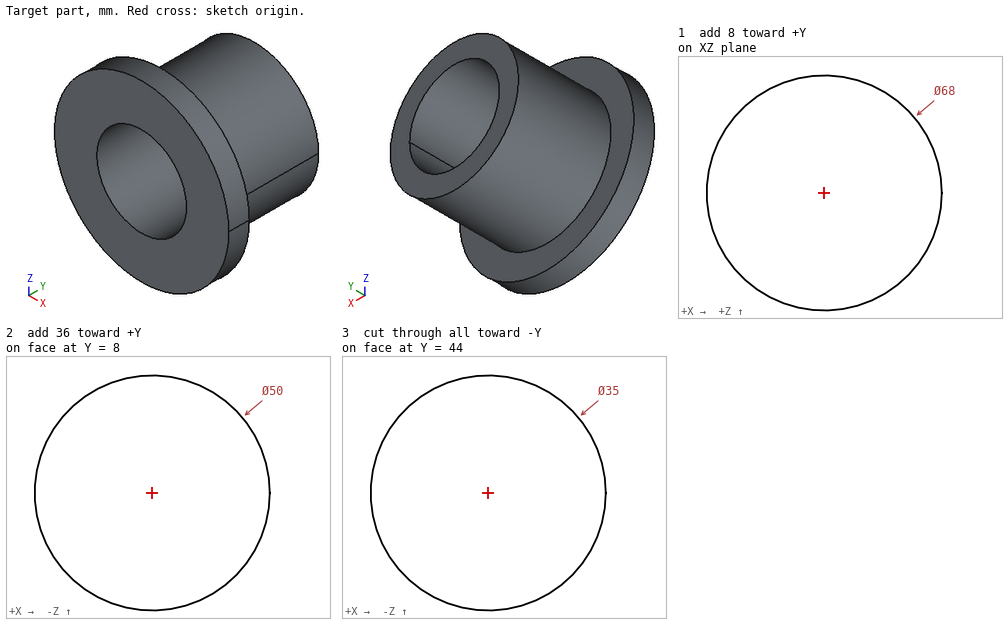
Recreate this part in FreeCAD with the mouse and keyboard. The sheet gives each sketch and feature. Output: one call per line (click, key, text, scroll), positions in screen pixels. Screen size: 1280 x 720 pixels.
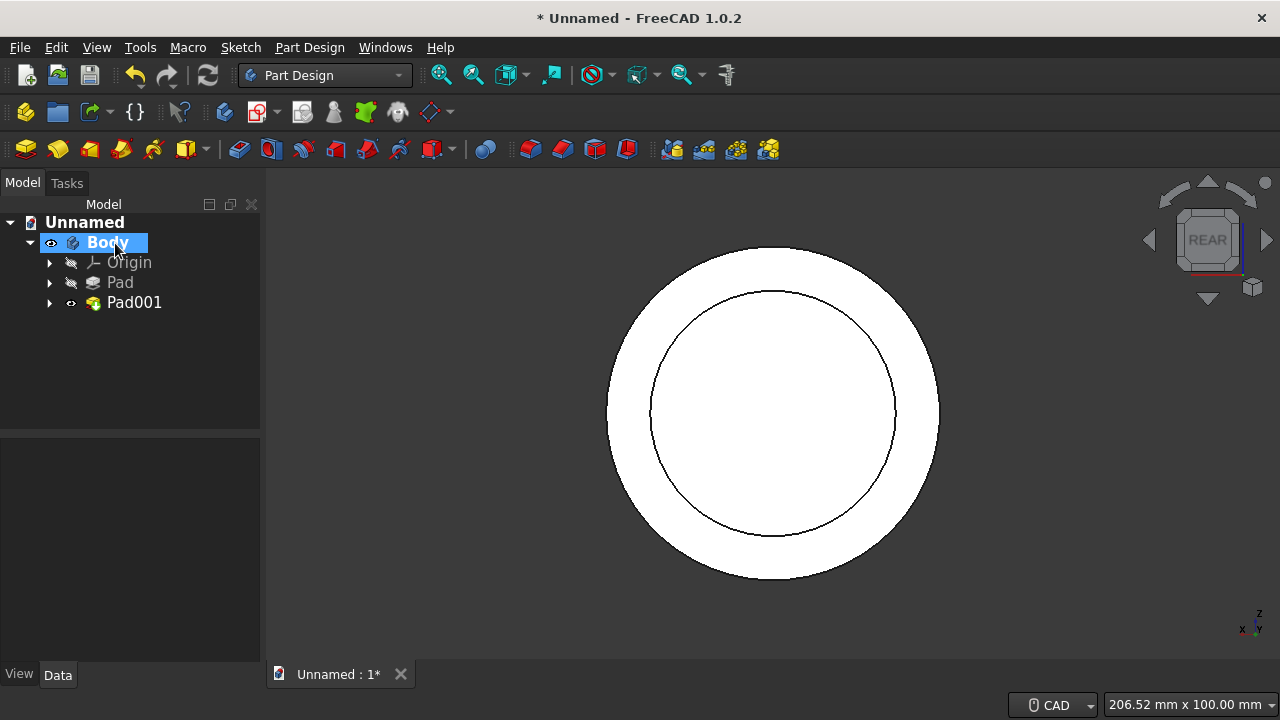
click(773, 412)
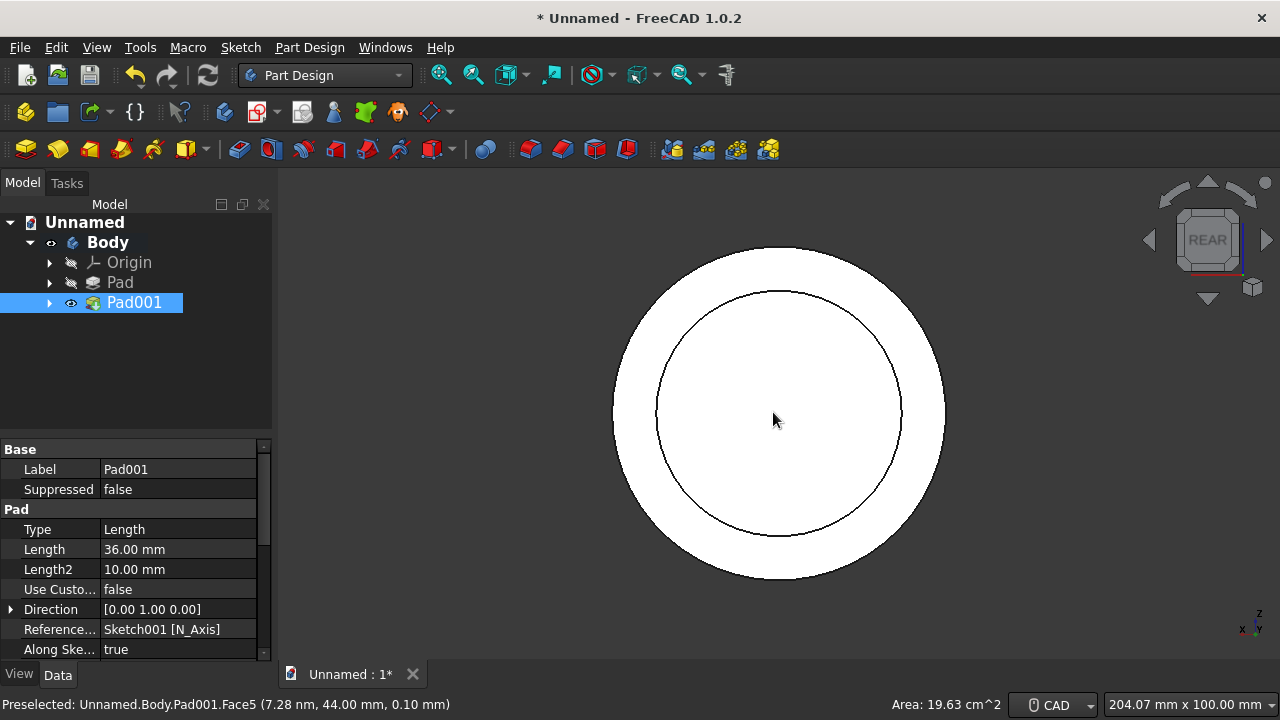
click(258, 112)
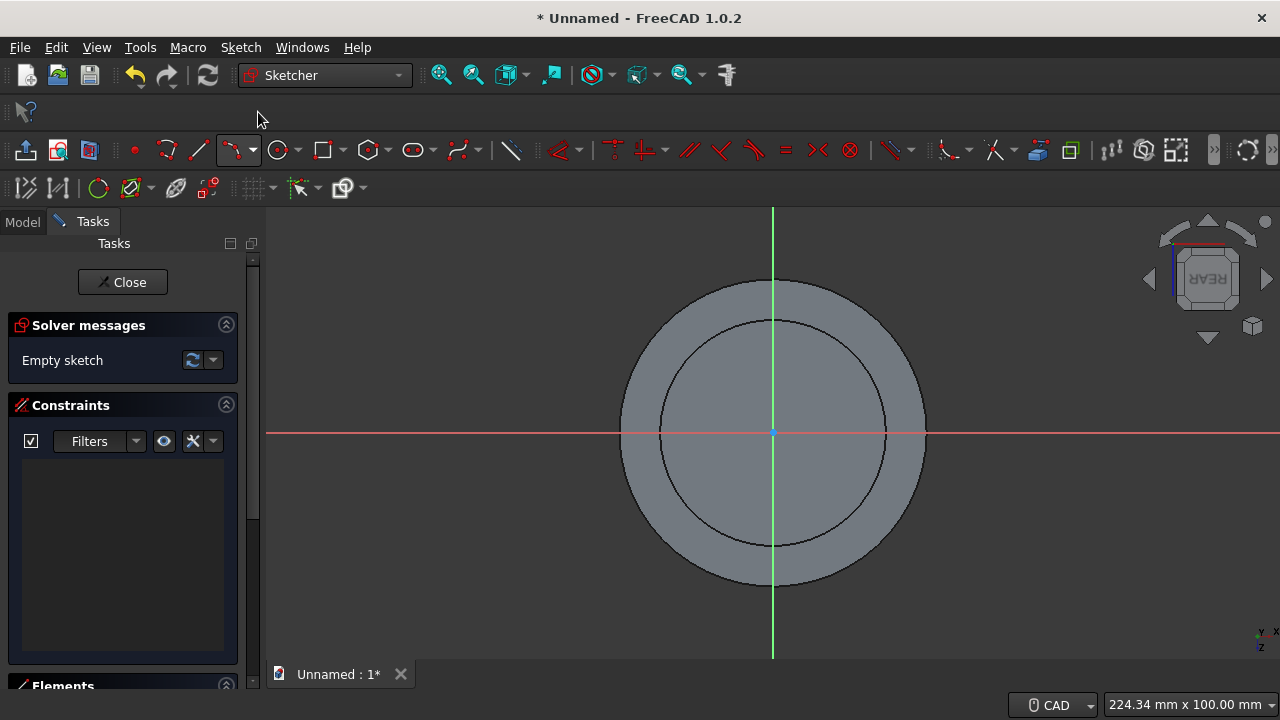
scroll(856, 433, up, 3)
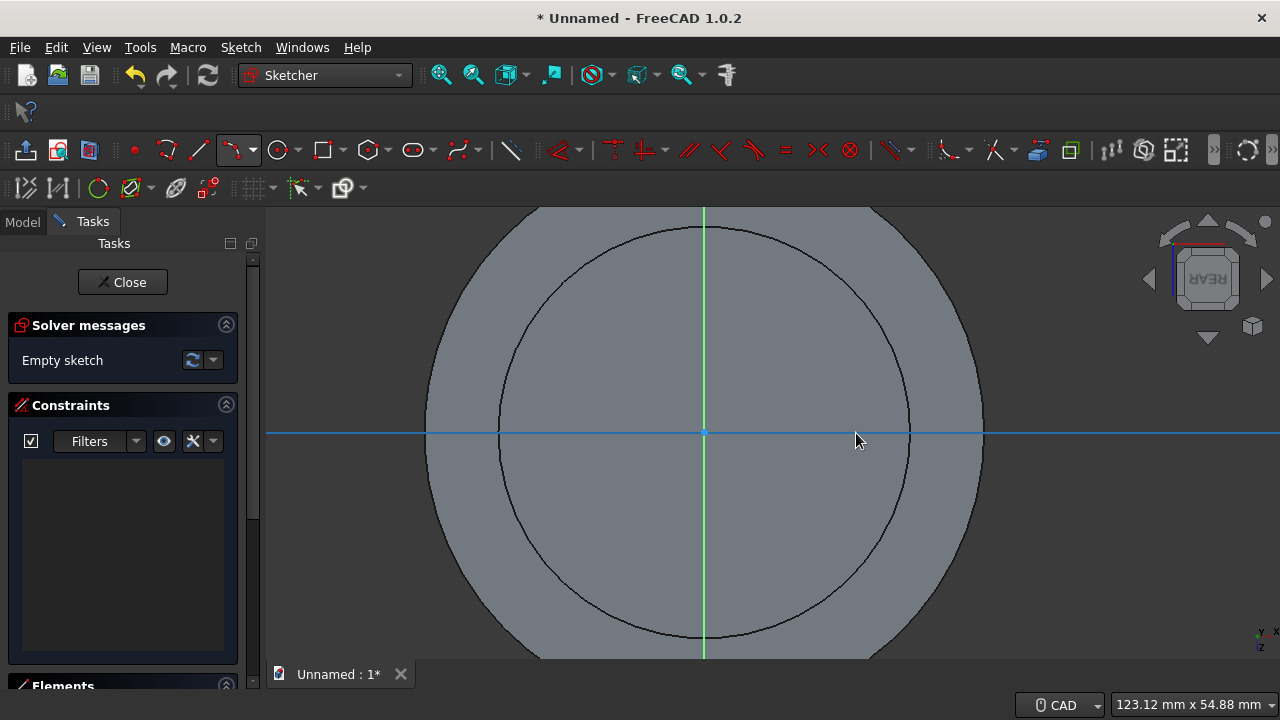
click(278, 150)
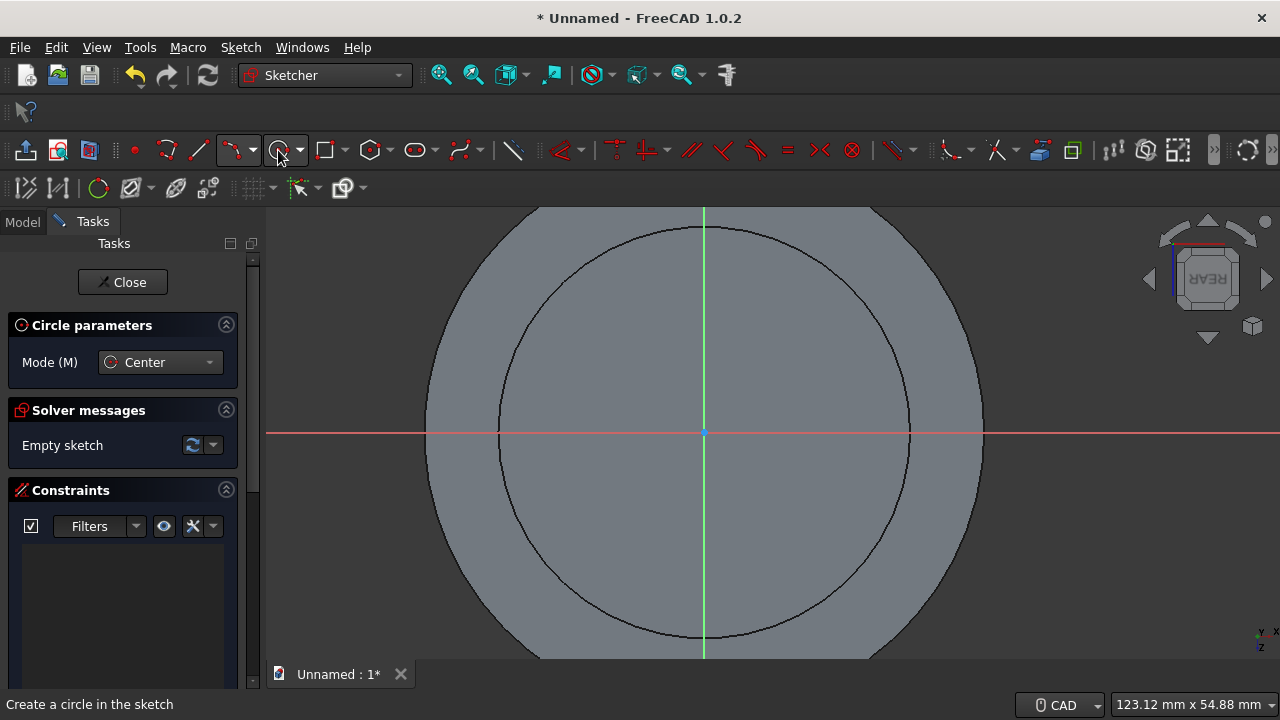
click(704, 433)
move(806, 331)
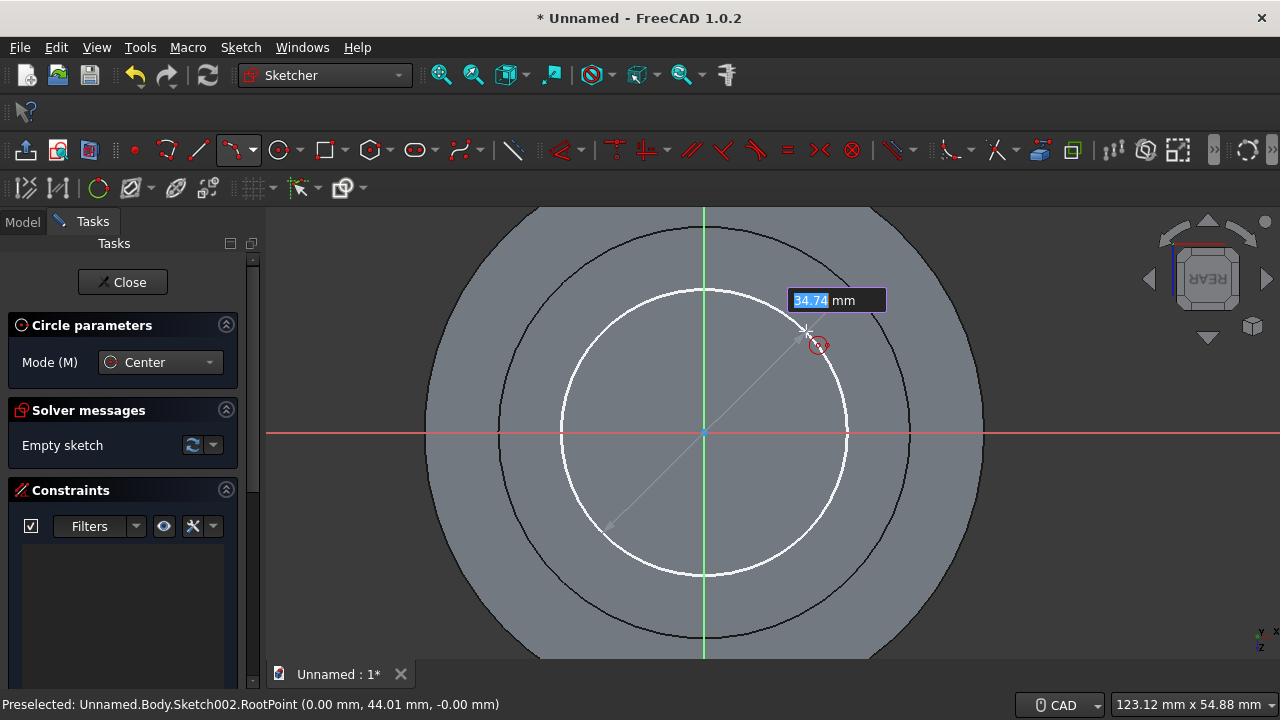
text(35)
key(Return)
key(Escape)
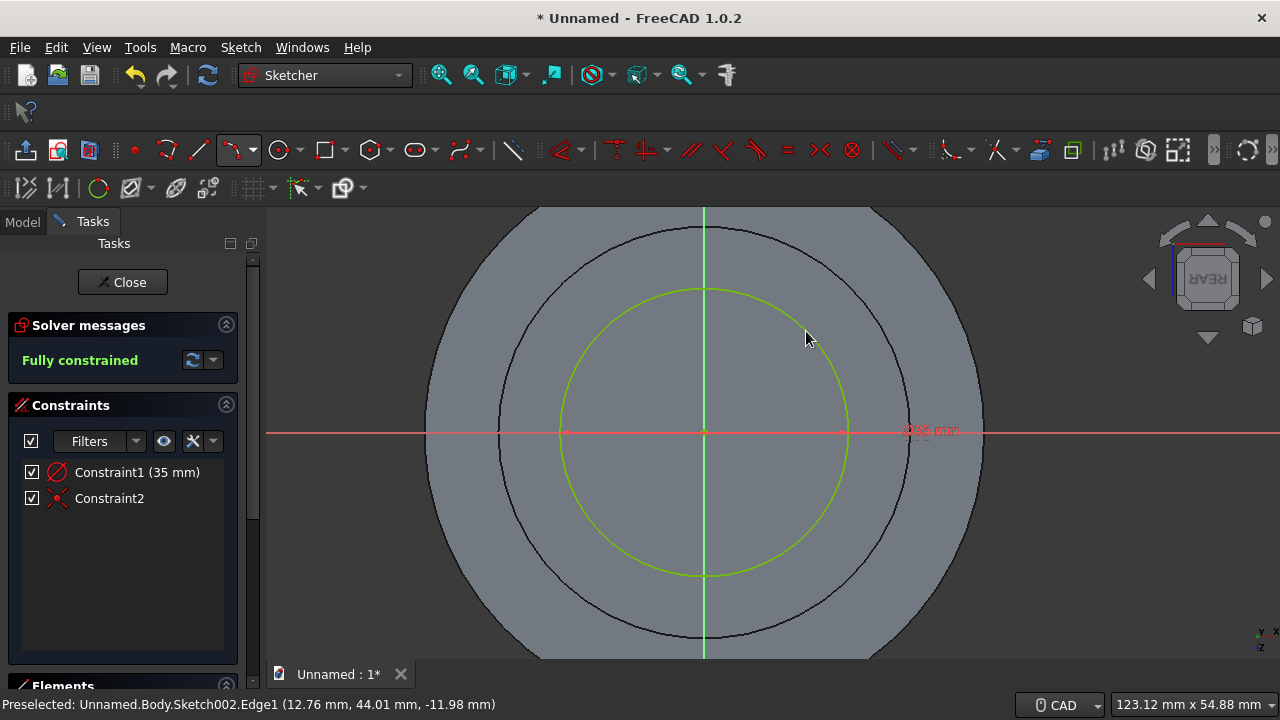
click(123, 282)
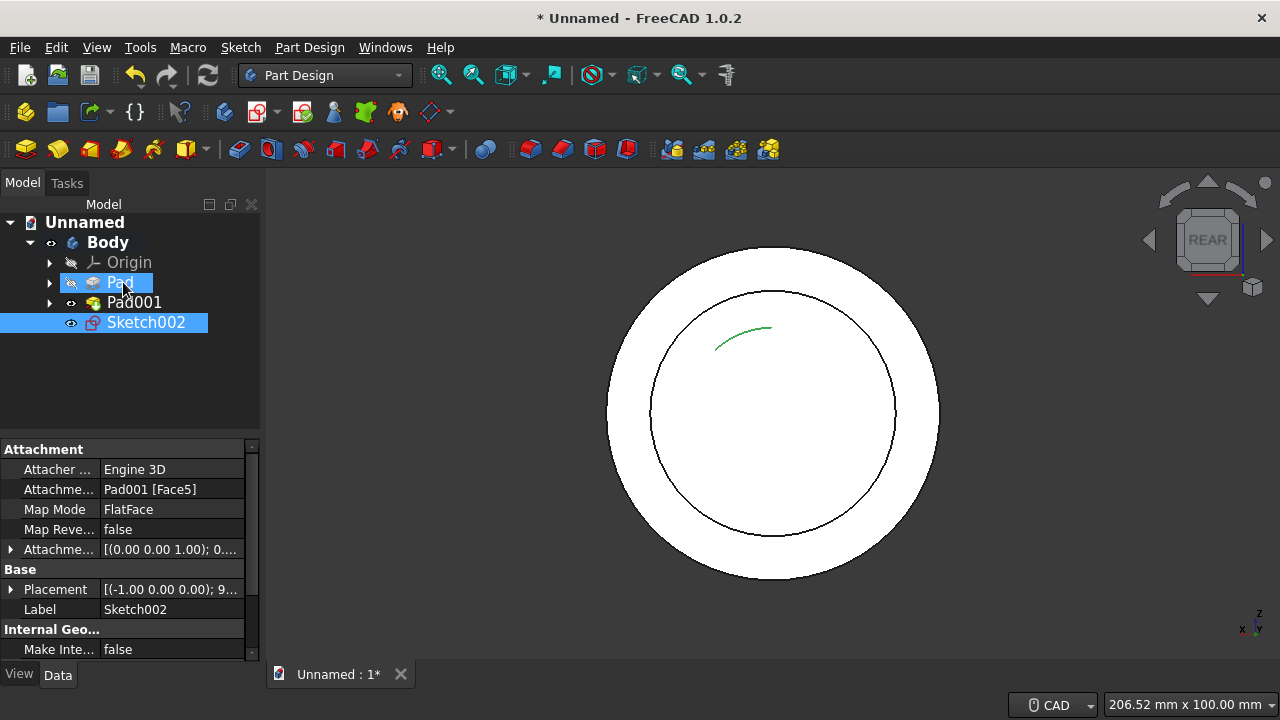
click(240, 150)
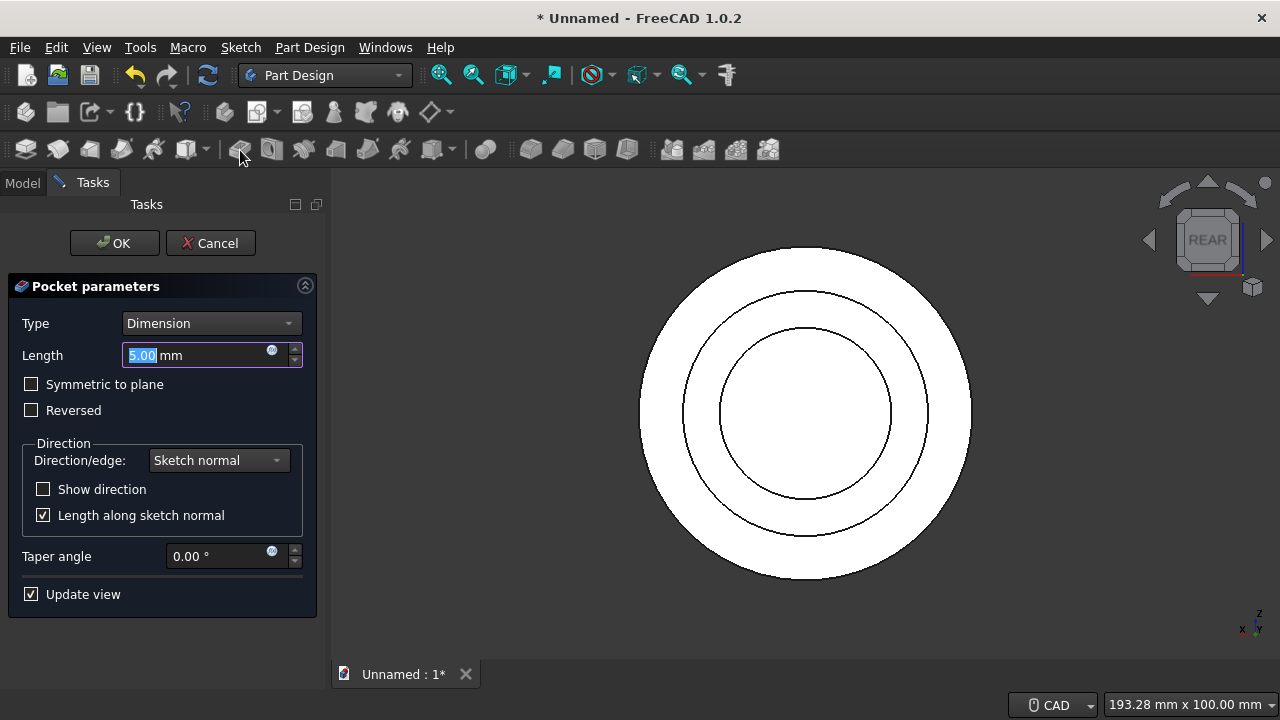
click(212, 324)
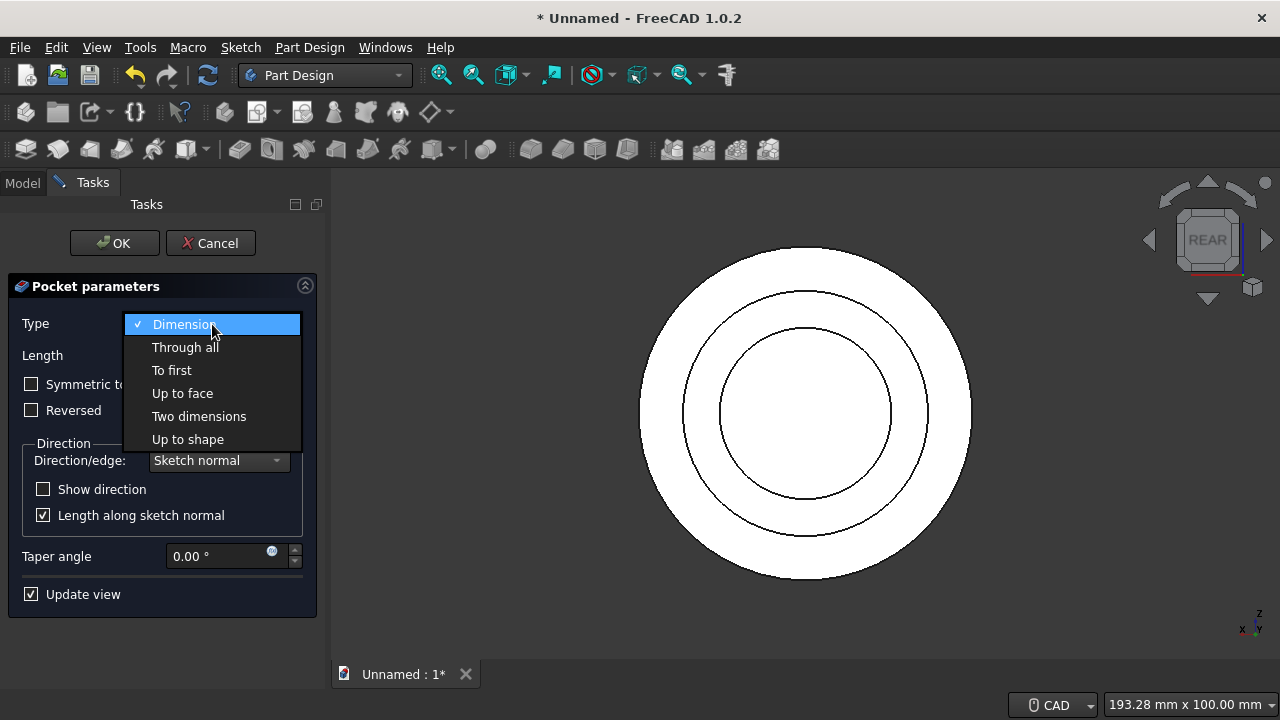
click(212, 348)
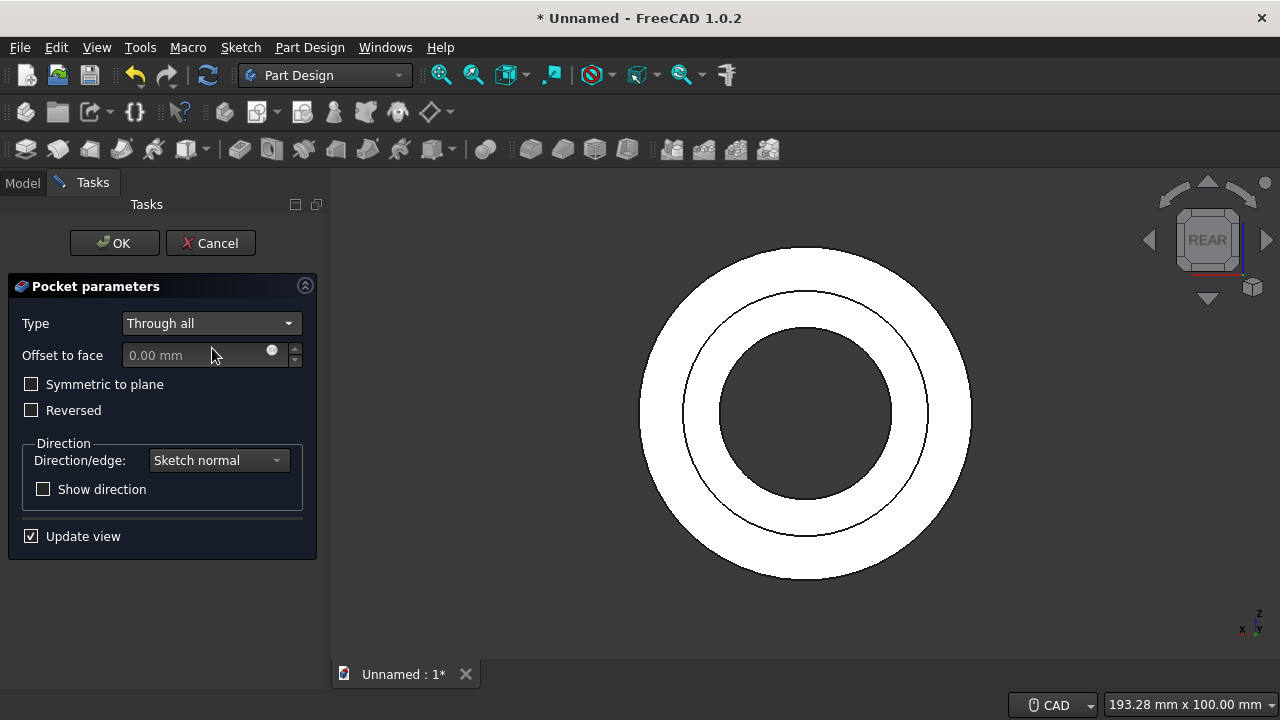
click(115, 243)